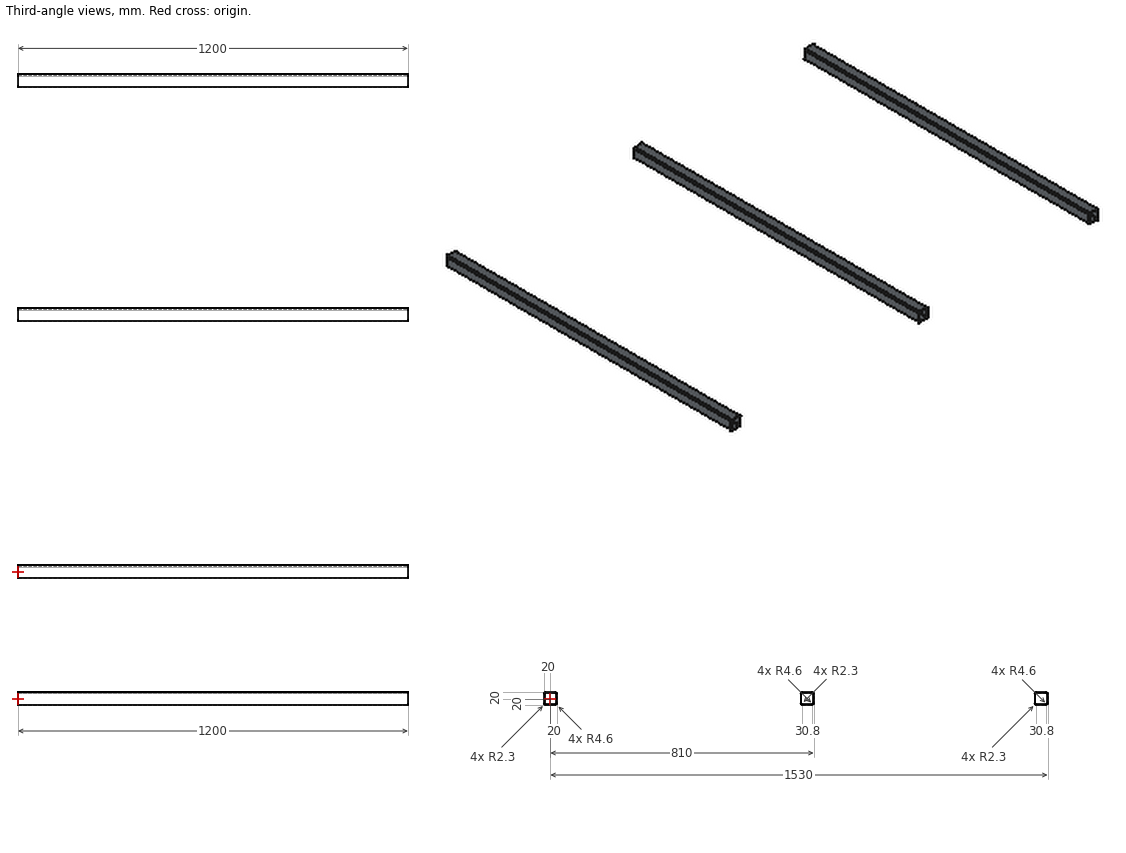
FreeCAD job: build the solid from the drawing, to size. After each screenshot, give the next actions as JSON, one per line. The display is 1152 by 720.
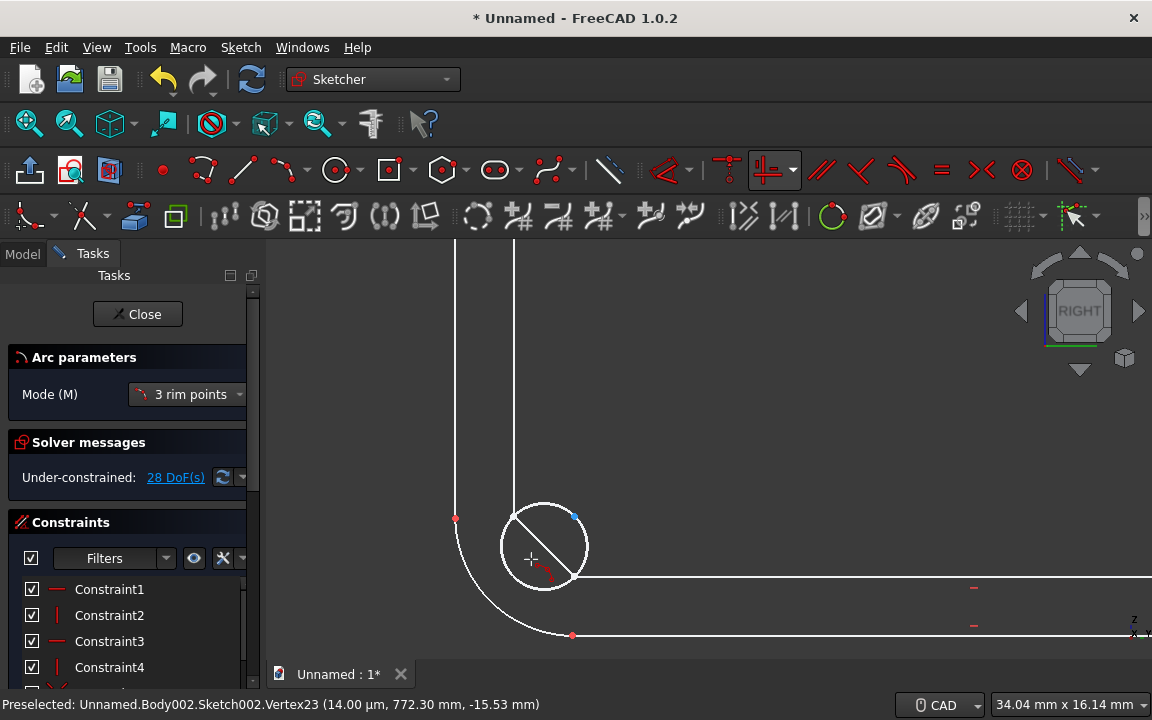
{"action": "left_click", "coordinate": [531, 555]}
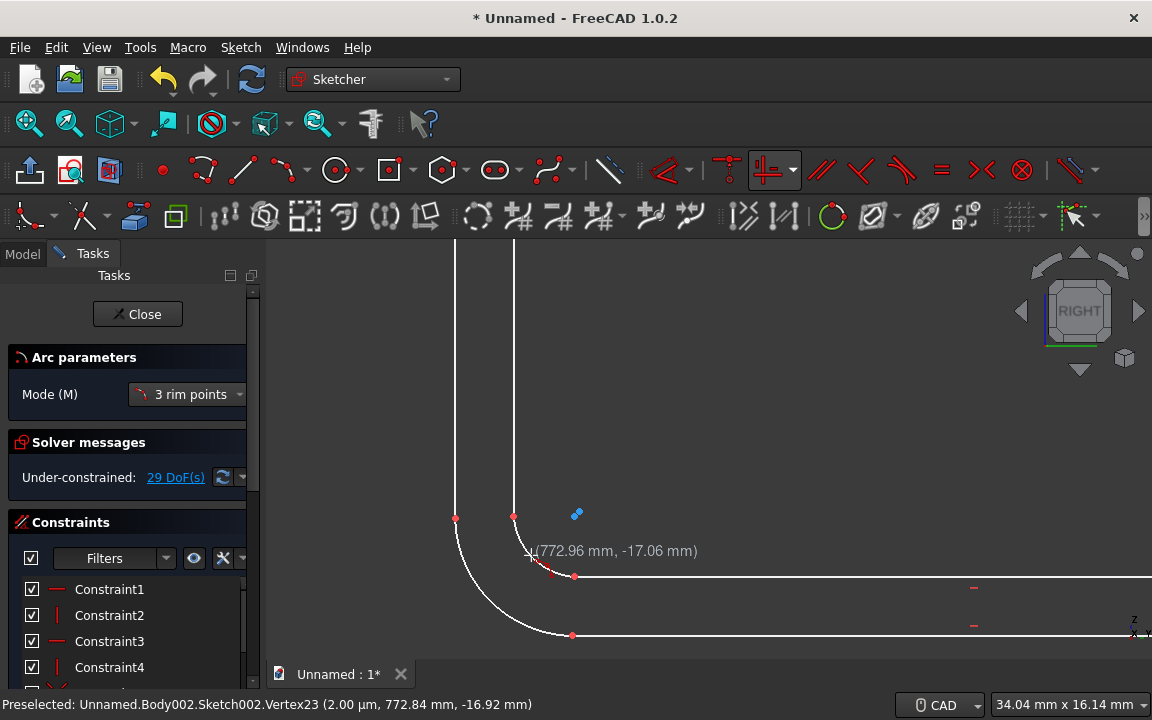
{"action": "scroll", "coordinate": [531, 559], "scroll_direction": "down", "scroll_amount": 7}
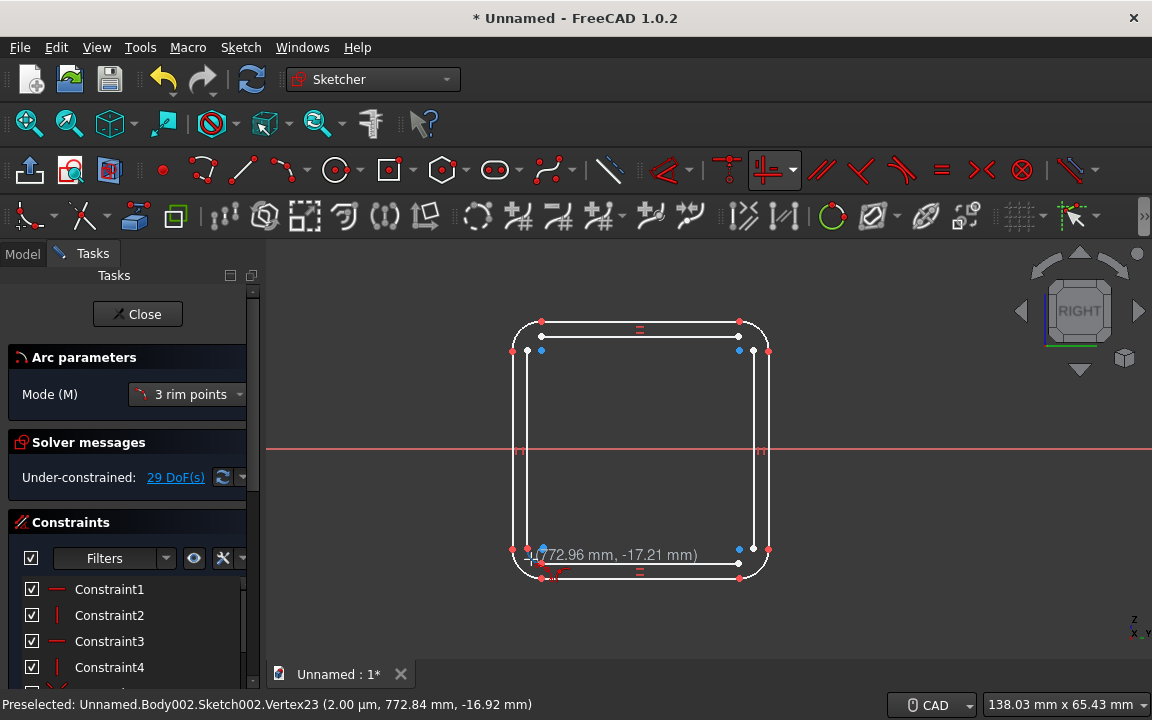
{"action": "left_click", "coordinate": [527, 351]}
{"action": "left_click", "coordinate": [542, 337]}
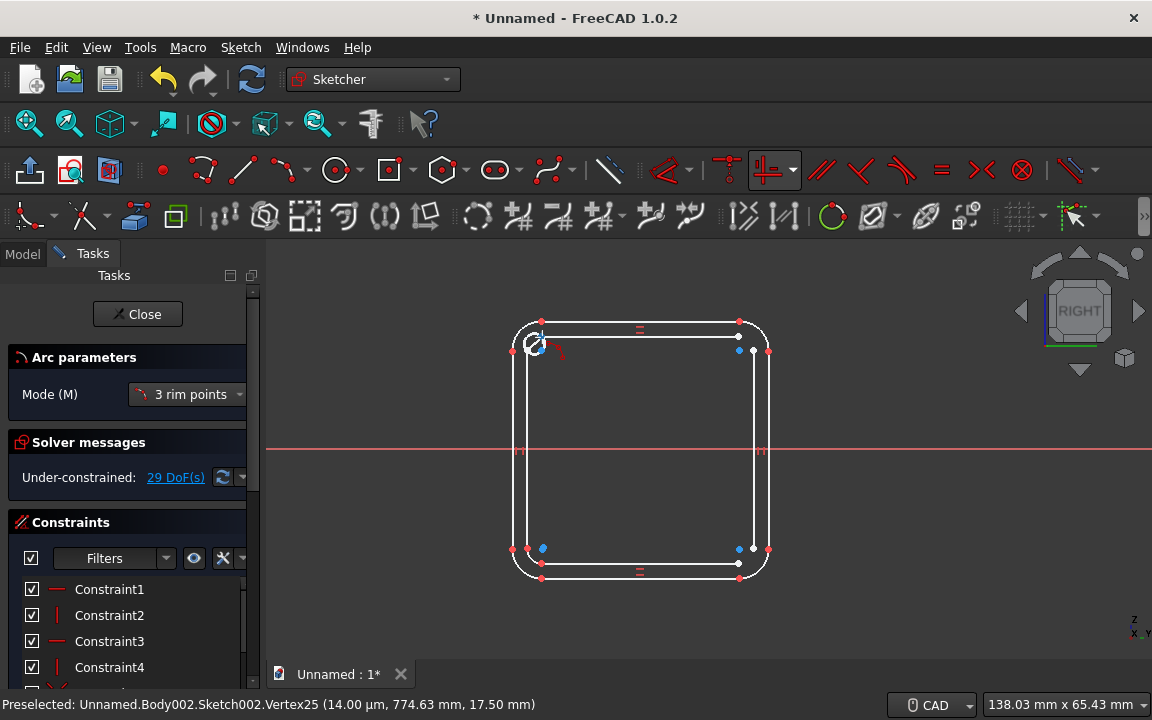
{"action": "scroll", "coordinate": [531, 340], "scroll_direction": "up", "scroll_amount": 7}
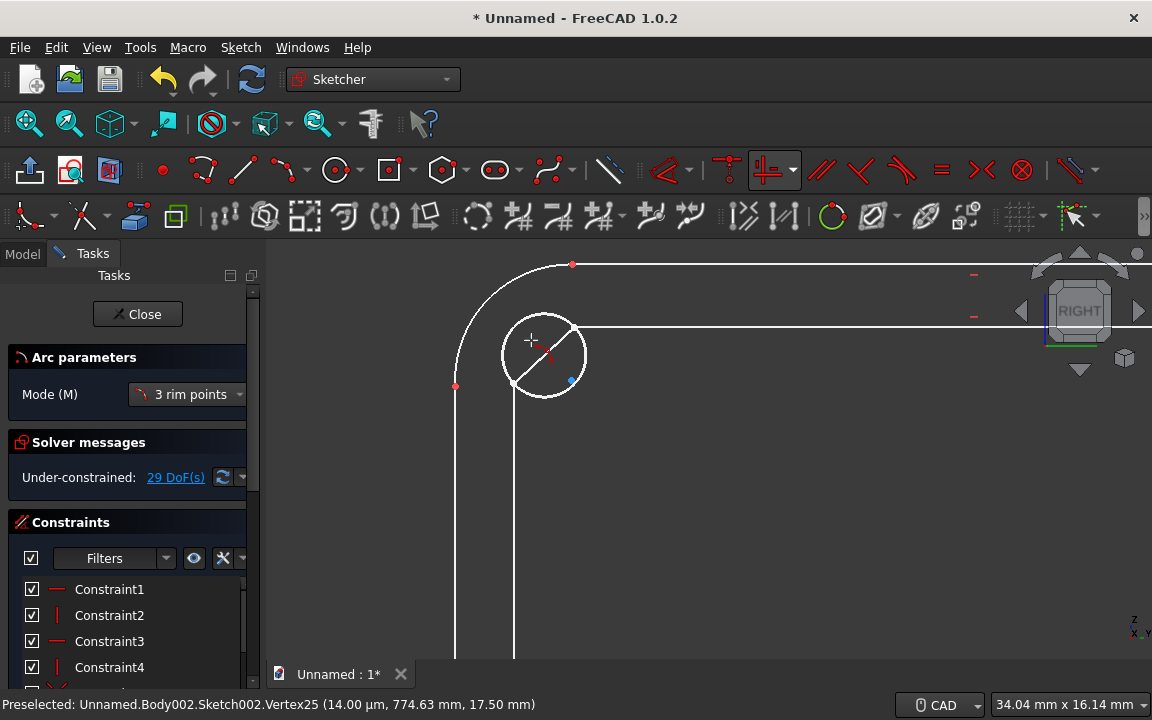
{"action": "left_click", "coordinate": [531, 339]}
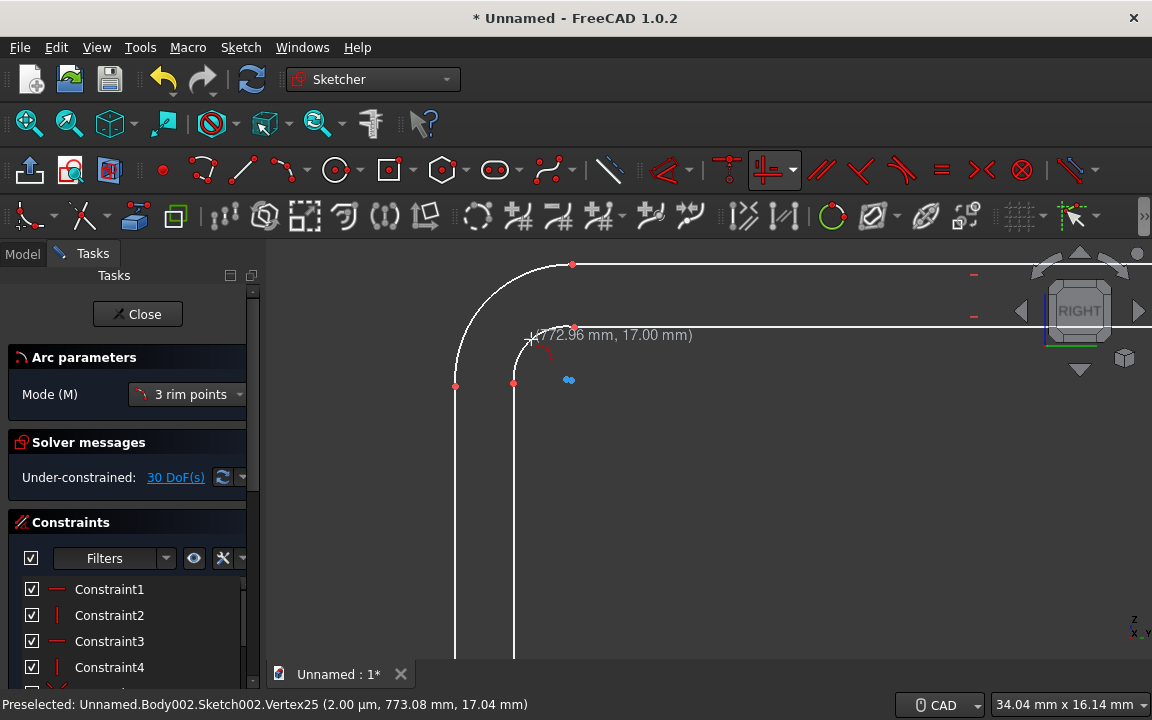
{"action": "scroll", "coordinate": [531, 340], "scroll_direction": "down", "scroll_amount": 7}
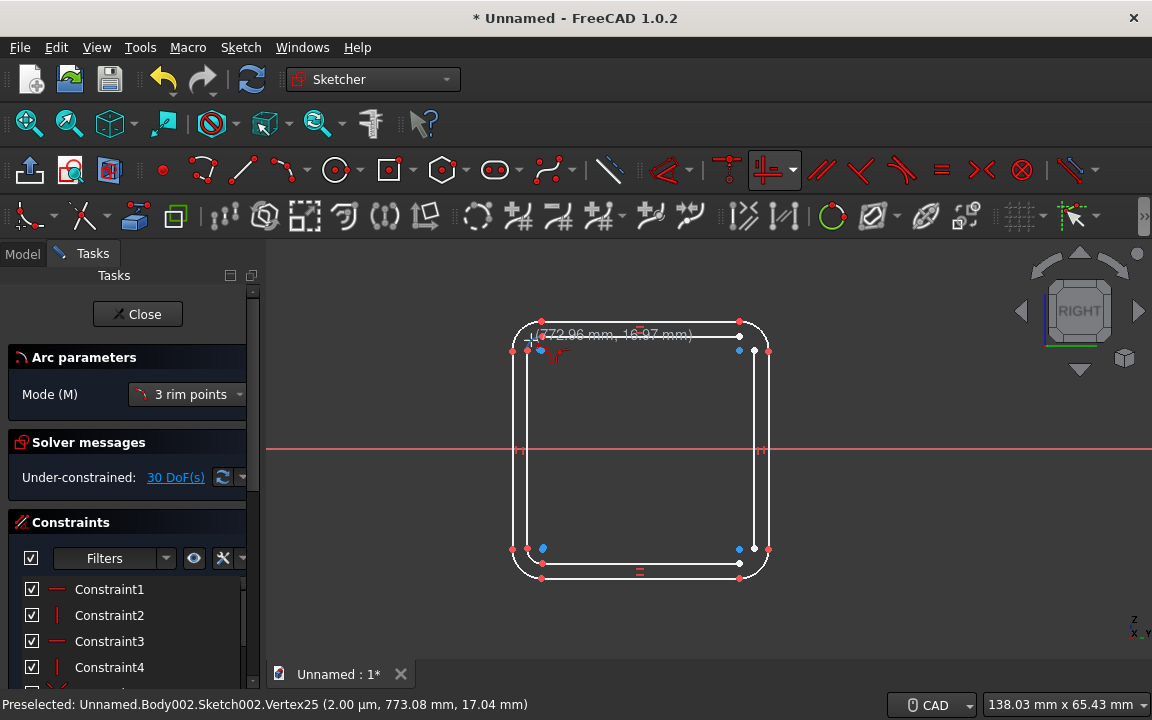
{"action": "left_click", "coordinate": [739, 337]}
{"action": "left_click", "coordinate": [754, 351]}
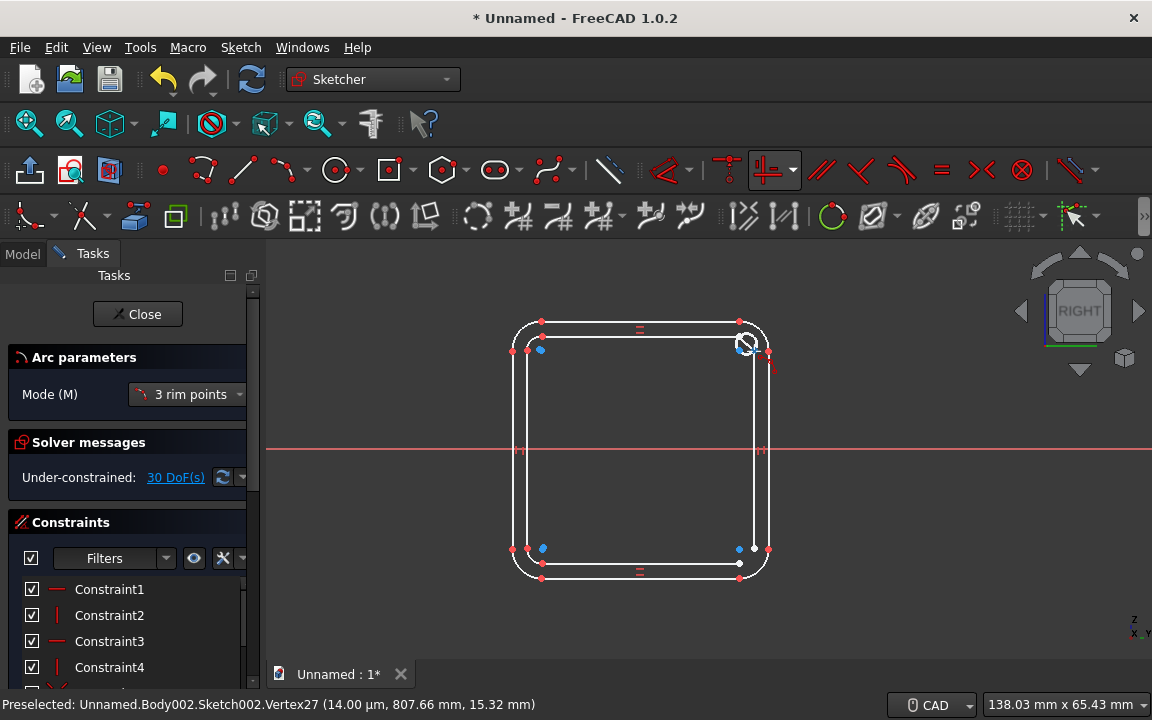
{"action": "scroll", "coordinate": [750, 340], "scroll_direction": "up", "scroll_amount": 7}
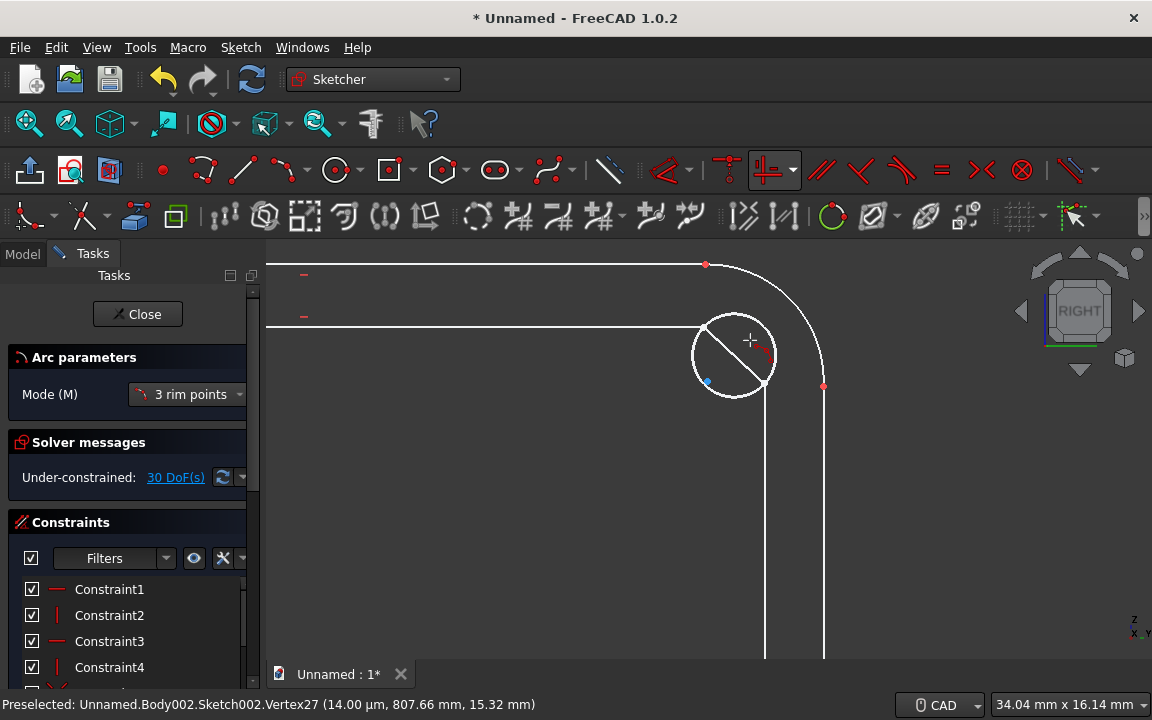
{"action": "left_click", "coordinate": [748, 339]}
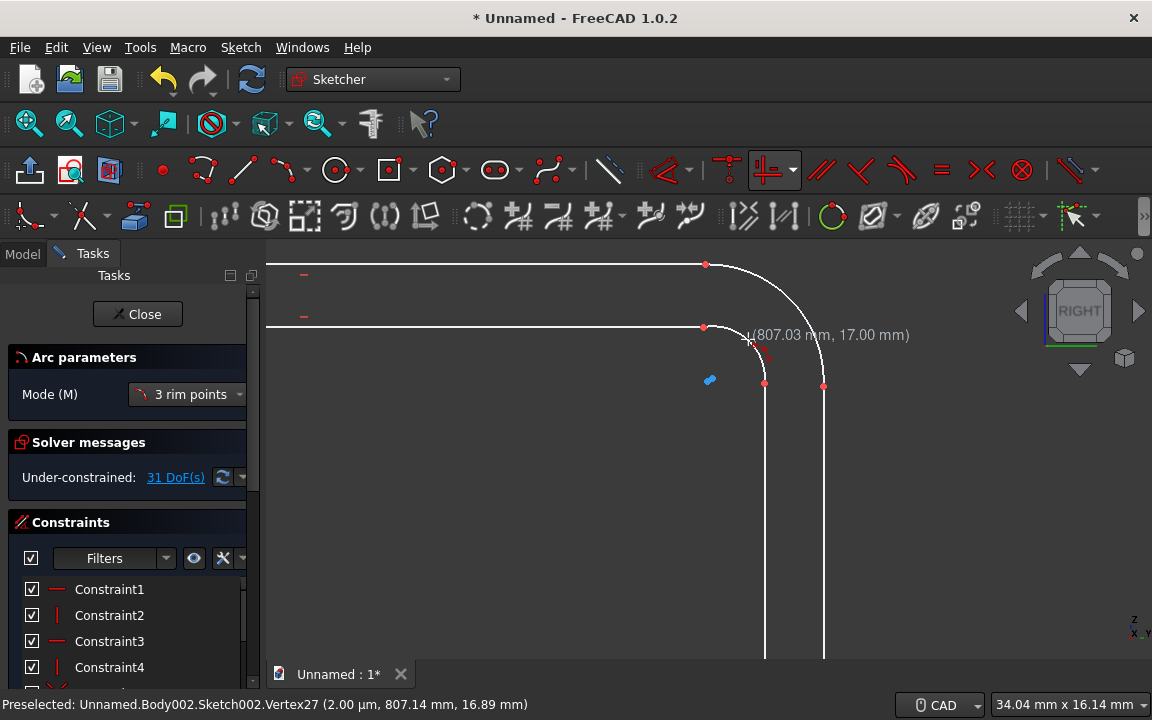
{"action": "scroll", "coordinate": [750, 340], "scroll_direction": "down", "scroll_amount": 7}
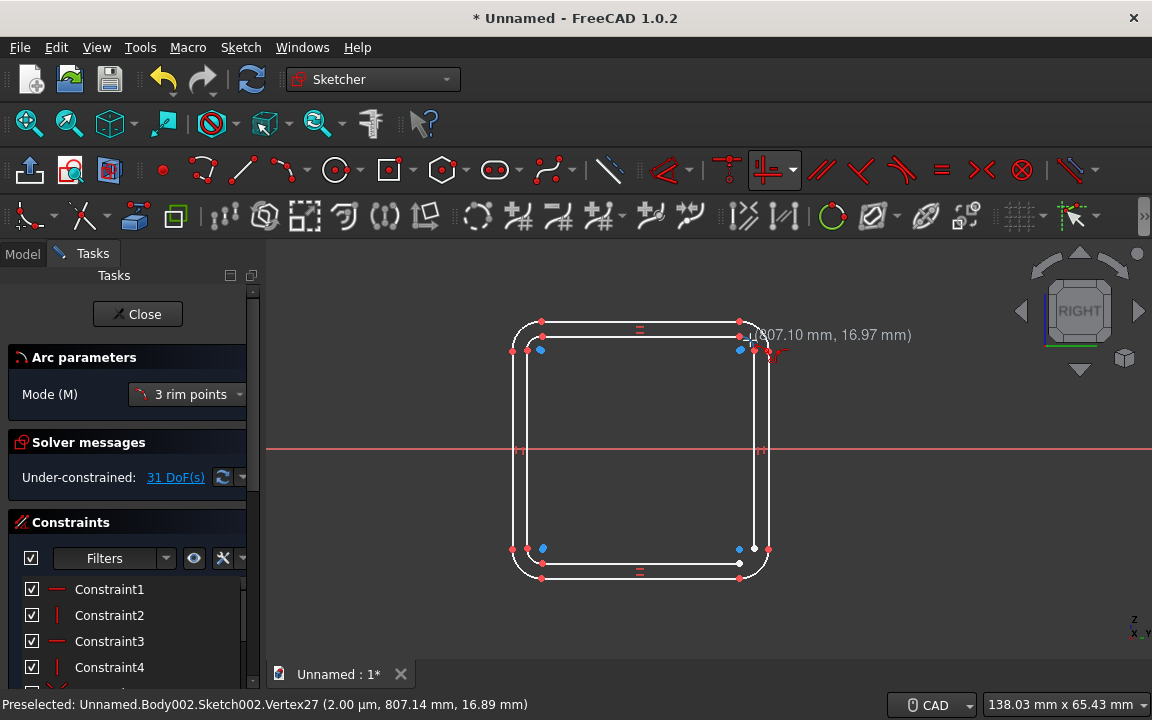
{"action": "left_click", "coordinate": [754, 549]}
{"action": "left_click", "coordinate": [739, 564]}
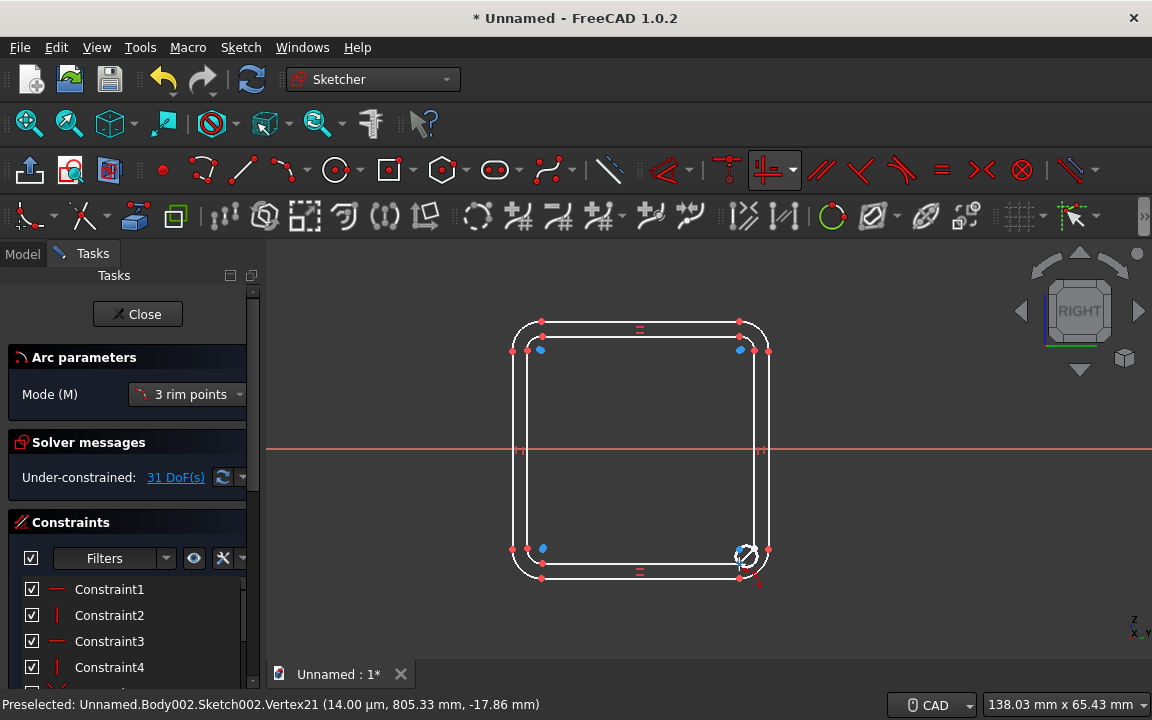
{"action": "scroll", "coordinate": [750, 559], "scroll_direction": "up", "scroll_amount": 7}